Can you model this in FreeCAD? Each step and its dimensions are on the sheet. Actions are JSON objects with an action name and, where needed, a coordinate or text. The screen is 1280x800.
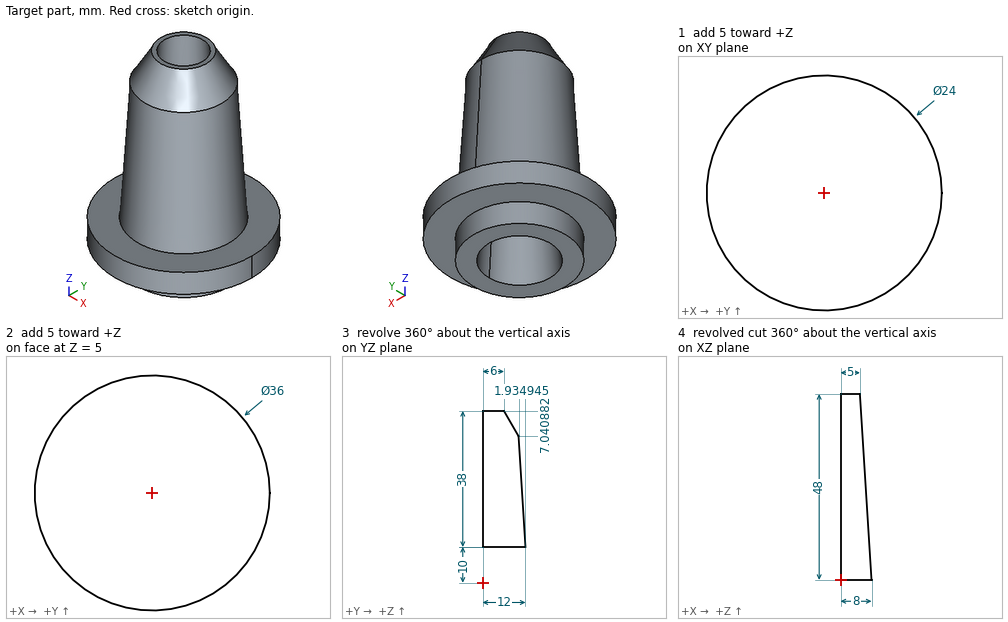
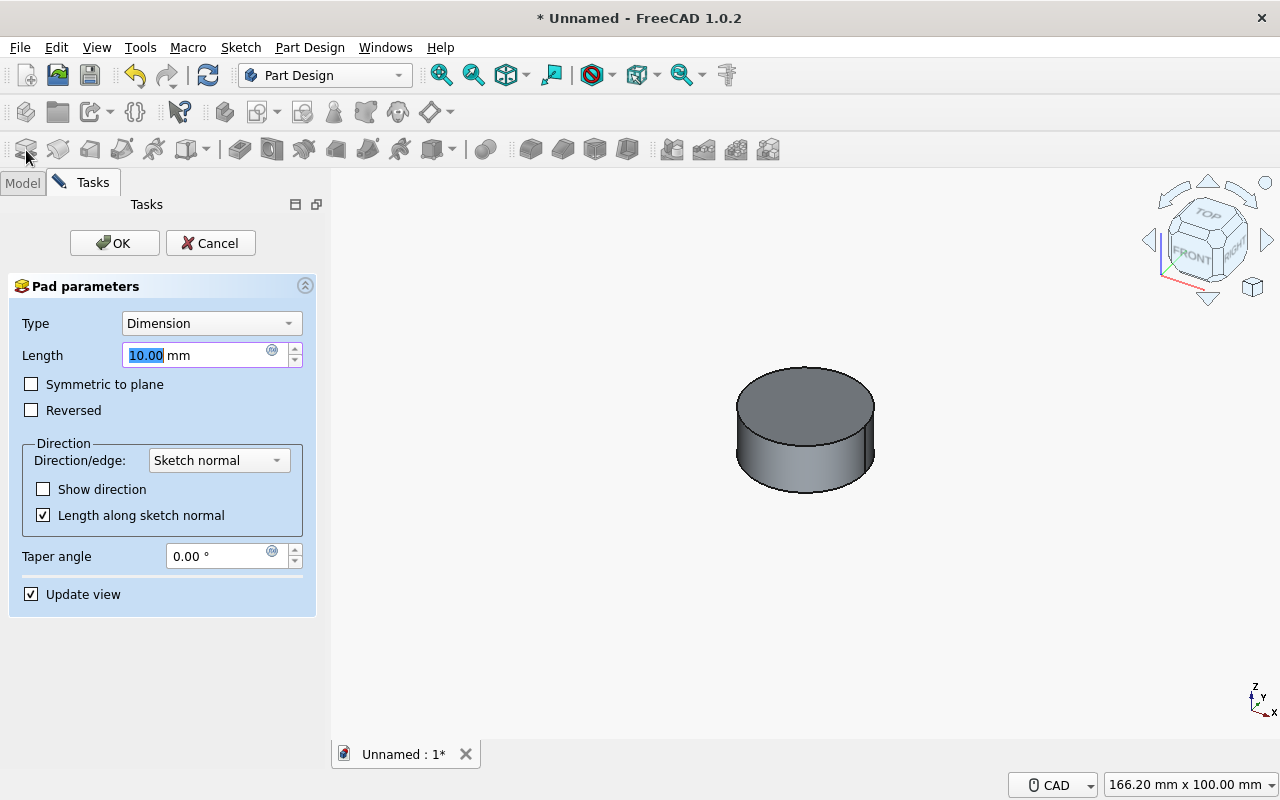
{"action": "type", "text": "5"}
{"action": "key", "text": "Tab"}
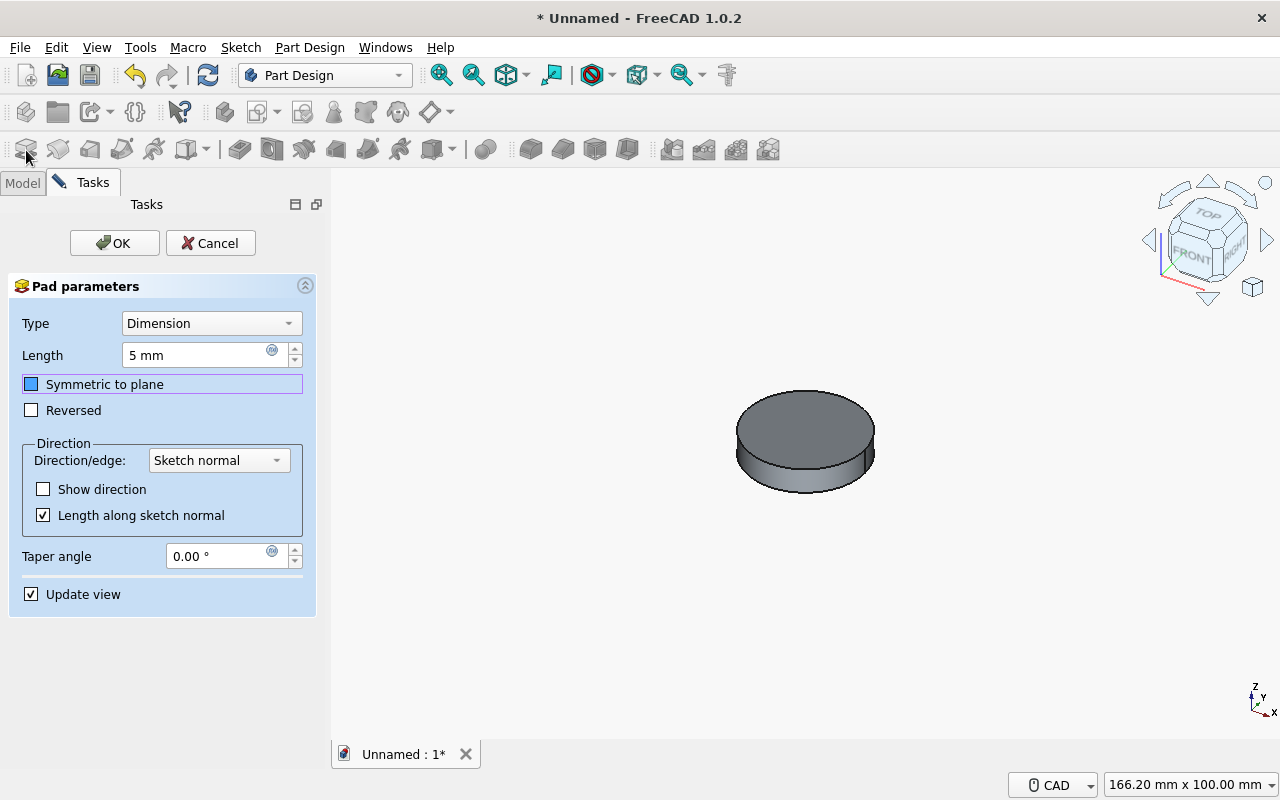
{"action": "left_click", "coordinate": [115, 243]}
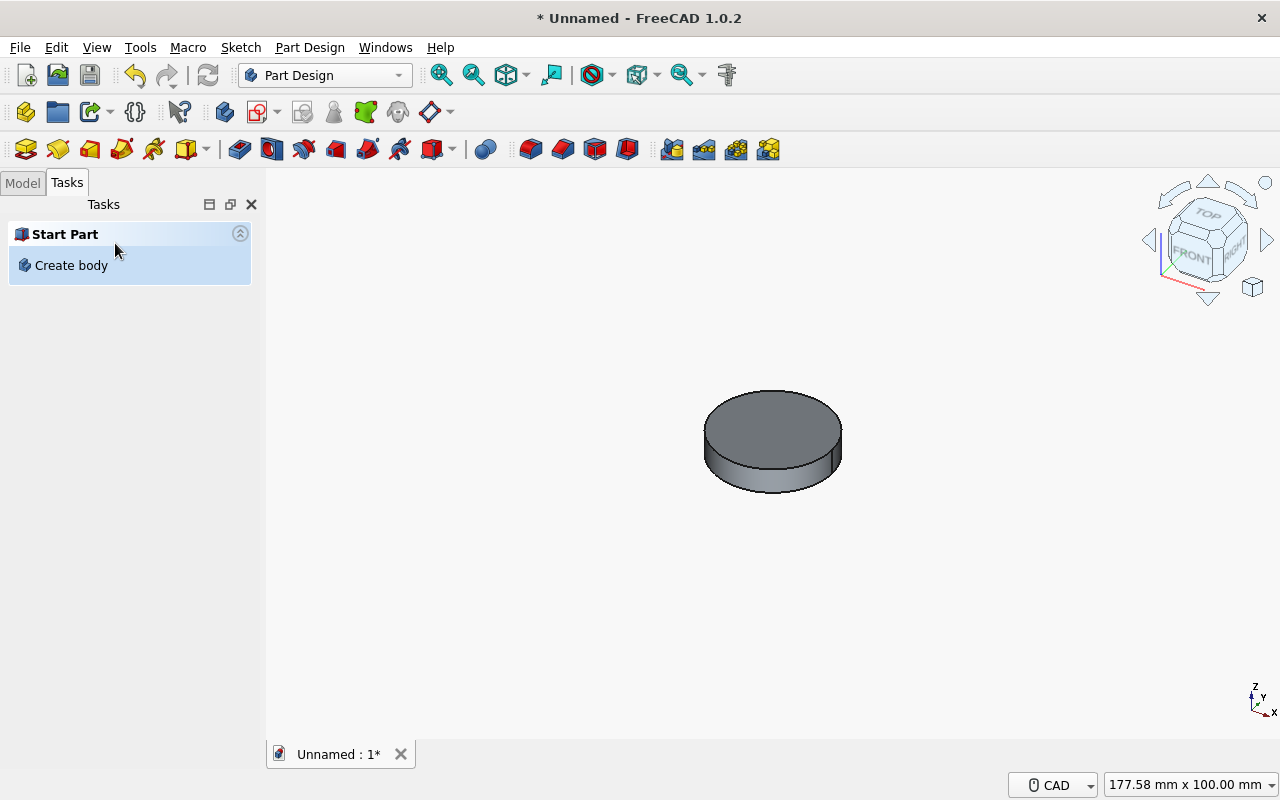
{"action": "left_click", "coordinate": [442, 76]}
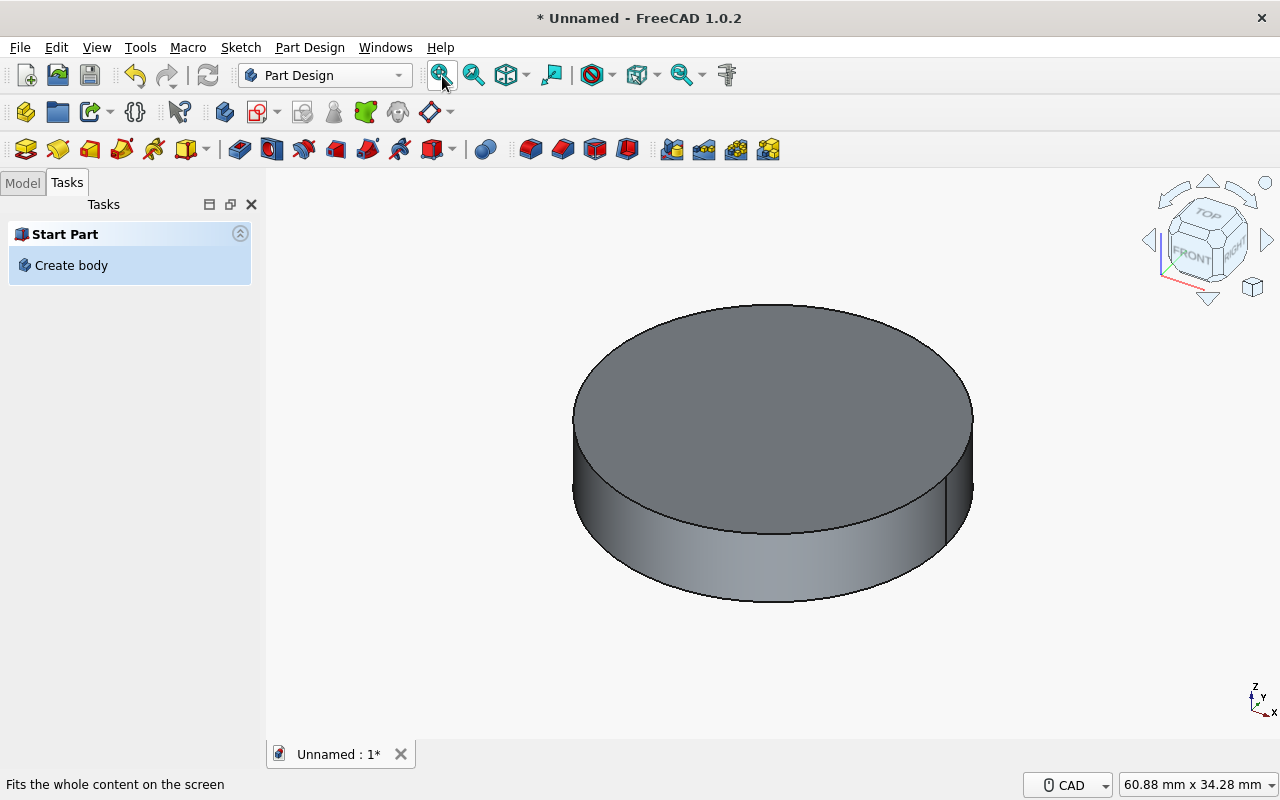
{"action": "left_click", "coordinate": [773, 418]}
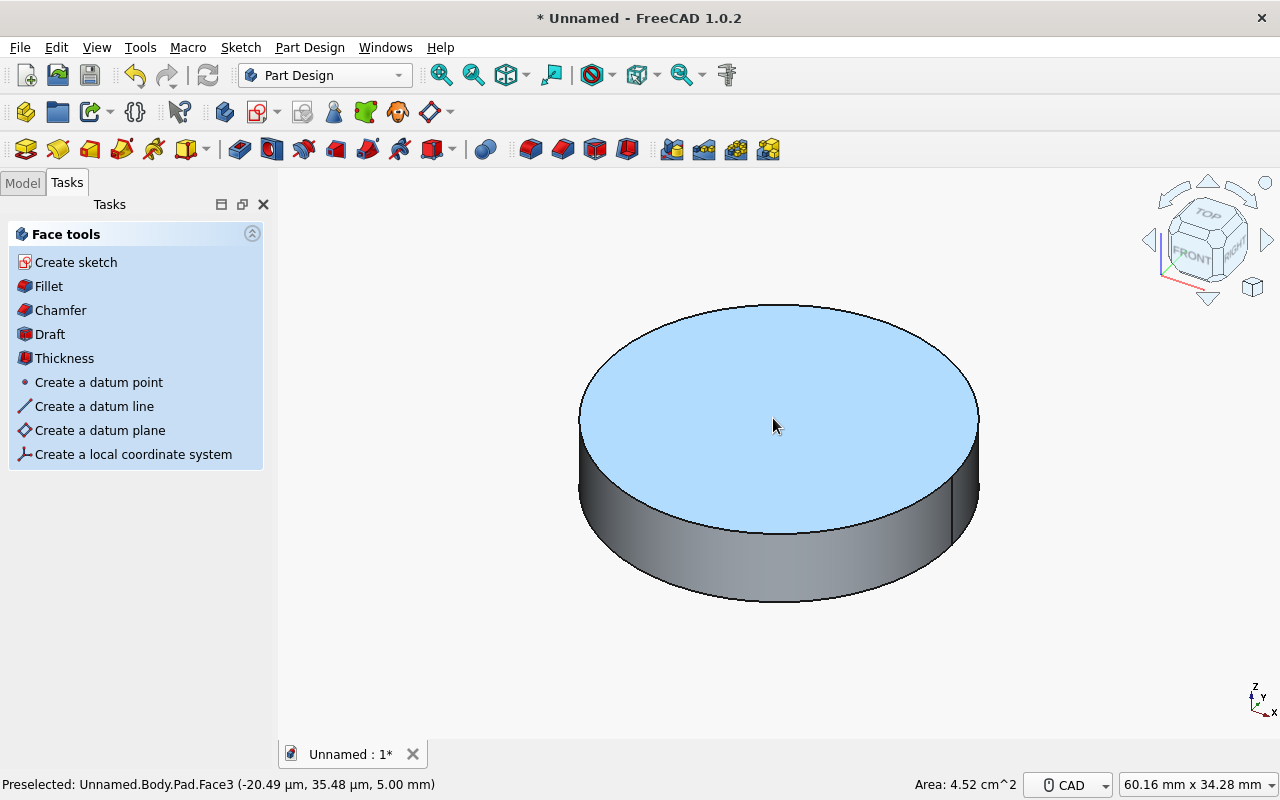
{"action": "left_click", "coordinate": [258, 112]}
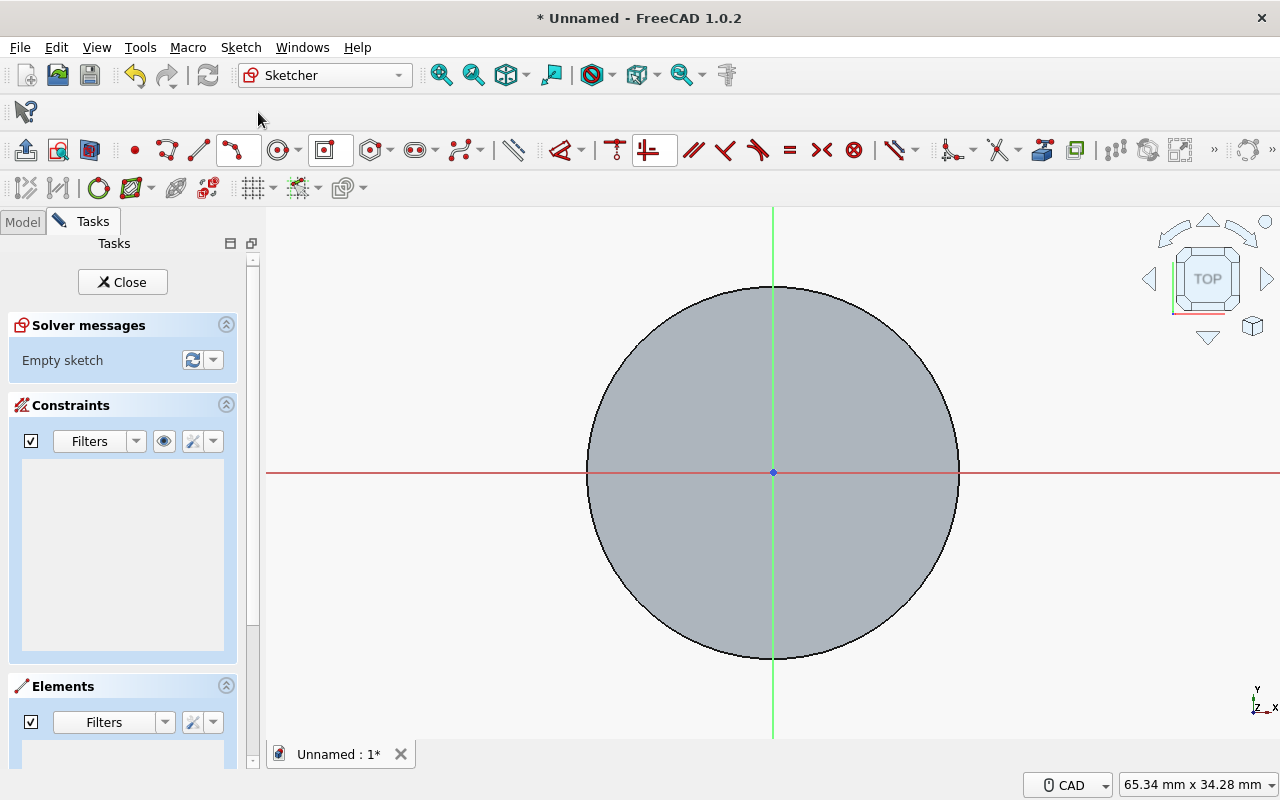
{"action": "scroll", "coordinate": [621, 473], "scroll_direction": "down", "scroll_amount": 3}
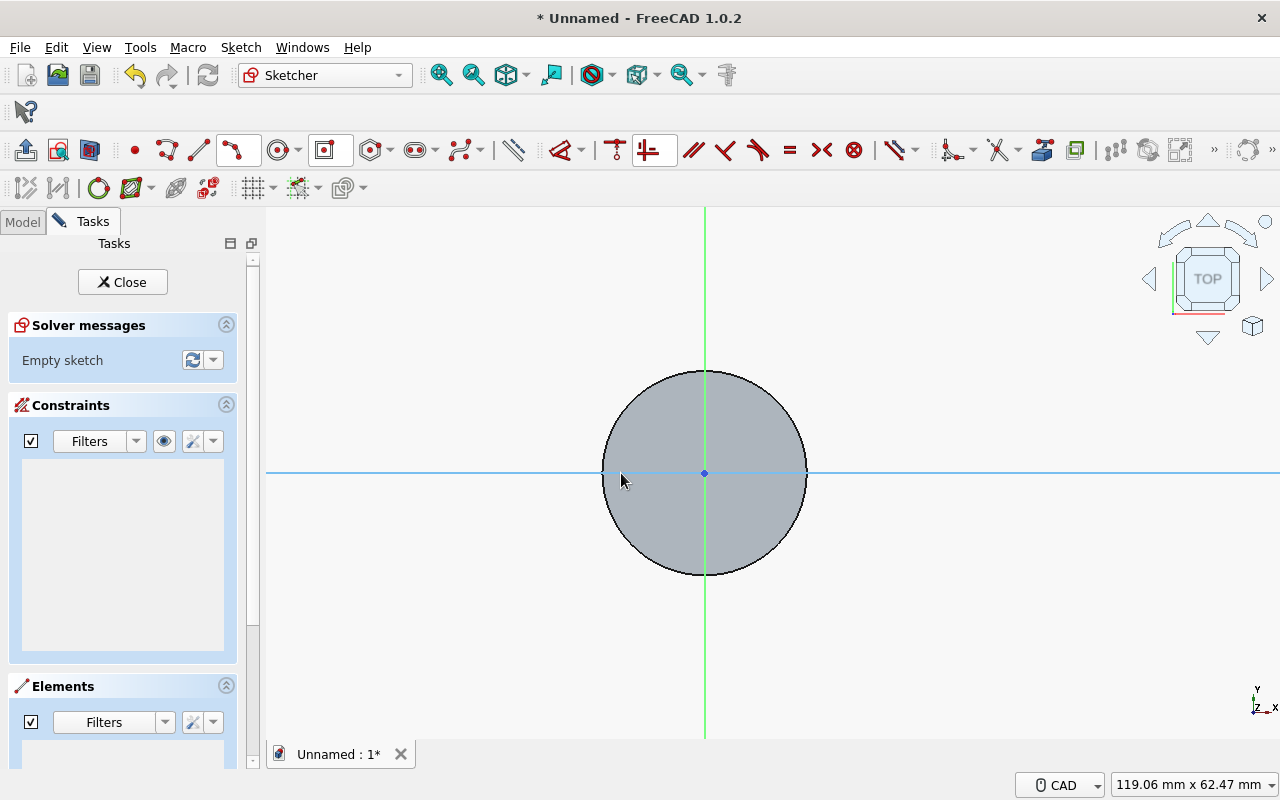
{"action": "left_click", "coordinate": [278, 150]}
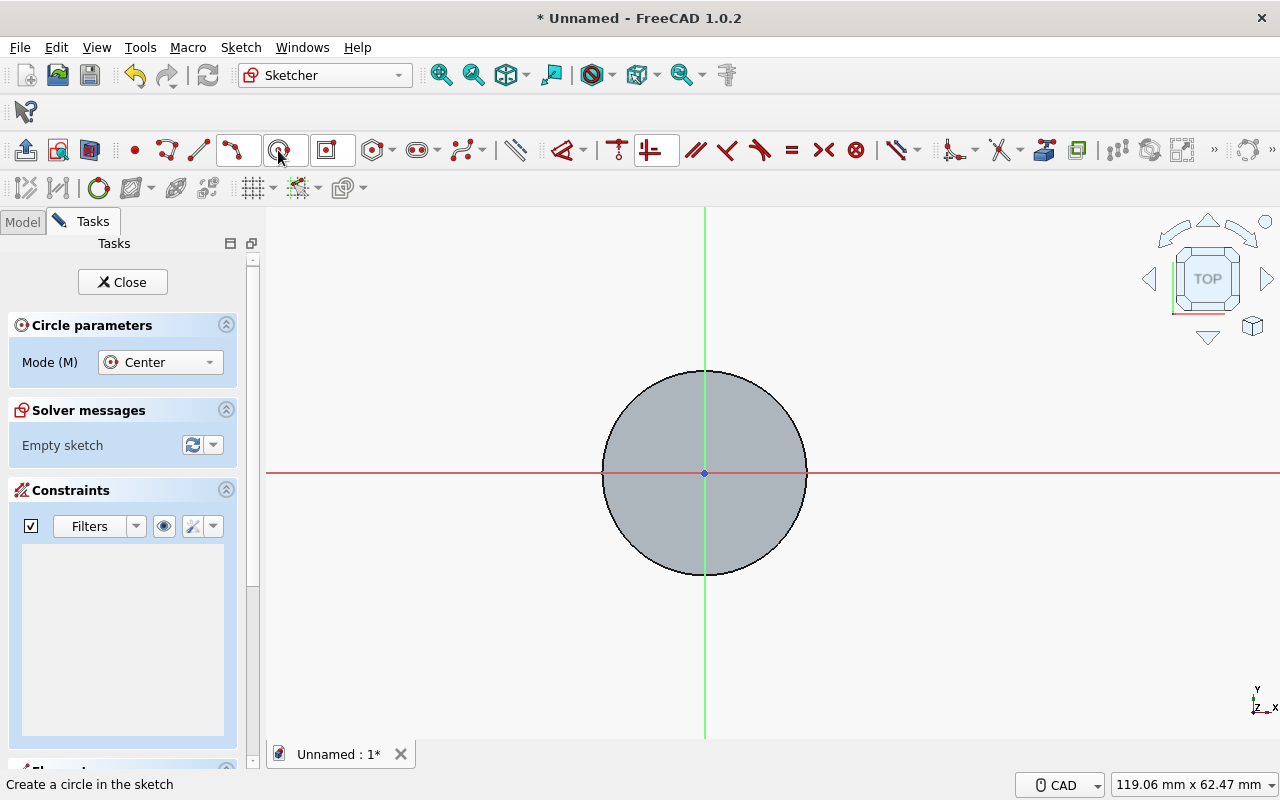
{"action": "left_click", "coordinate": [705, 473]}
{"action": "mouse_move", "coordinate": [813, 365]}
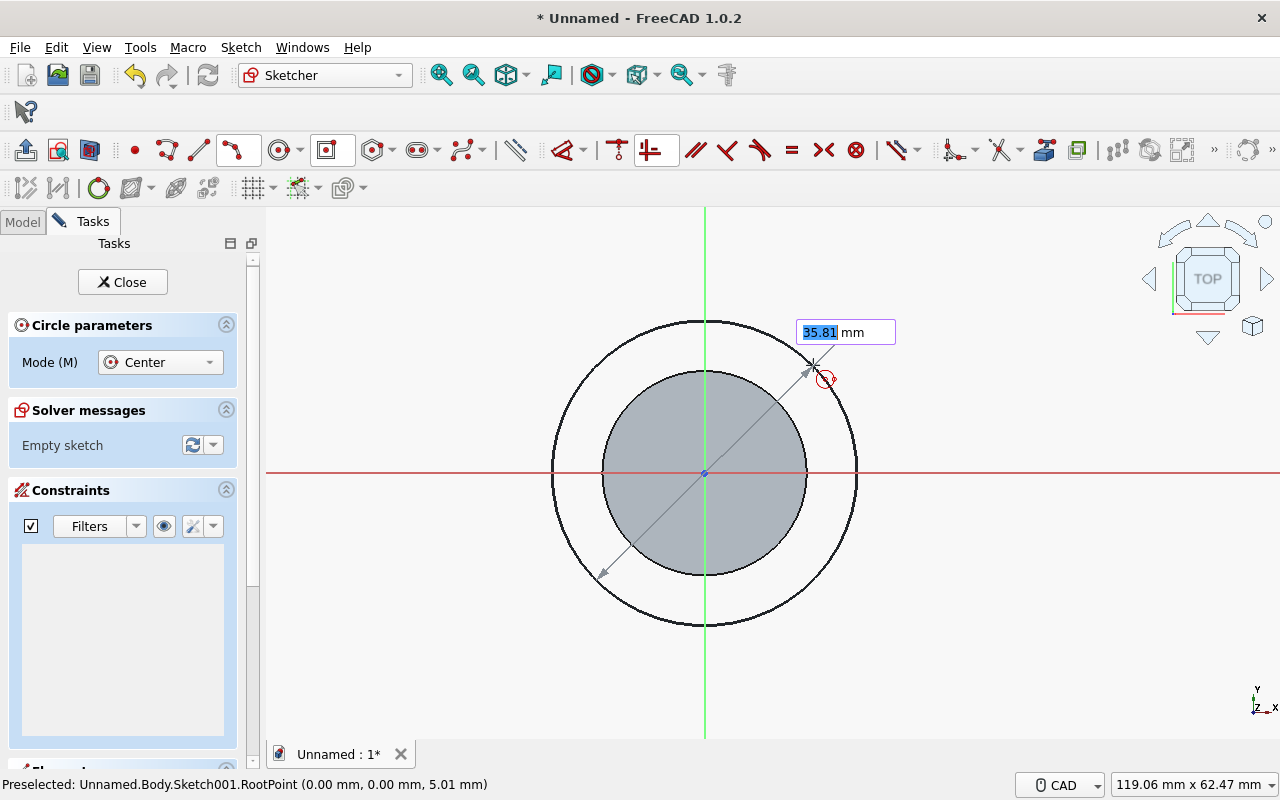
{"action": "type", "text": "36"}
{"action": "key", "text": "Return"}
{"action": "key", "text": "Escape"}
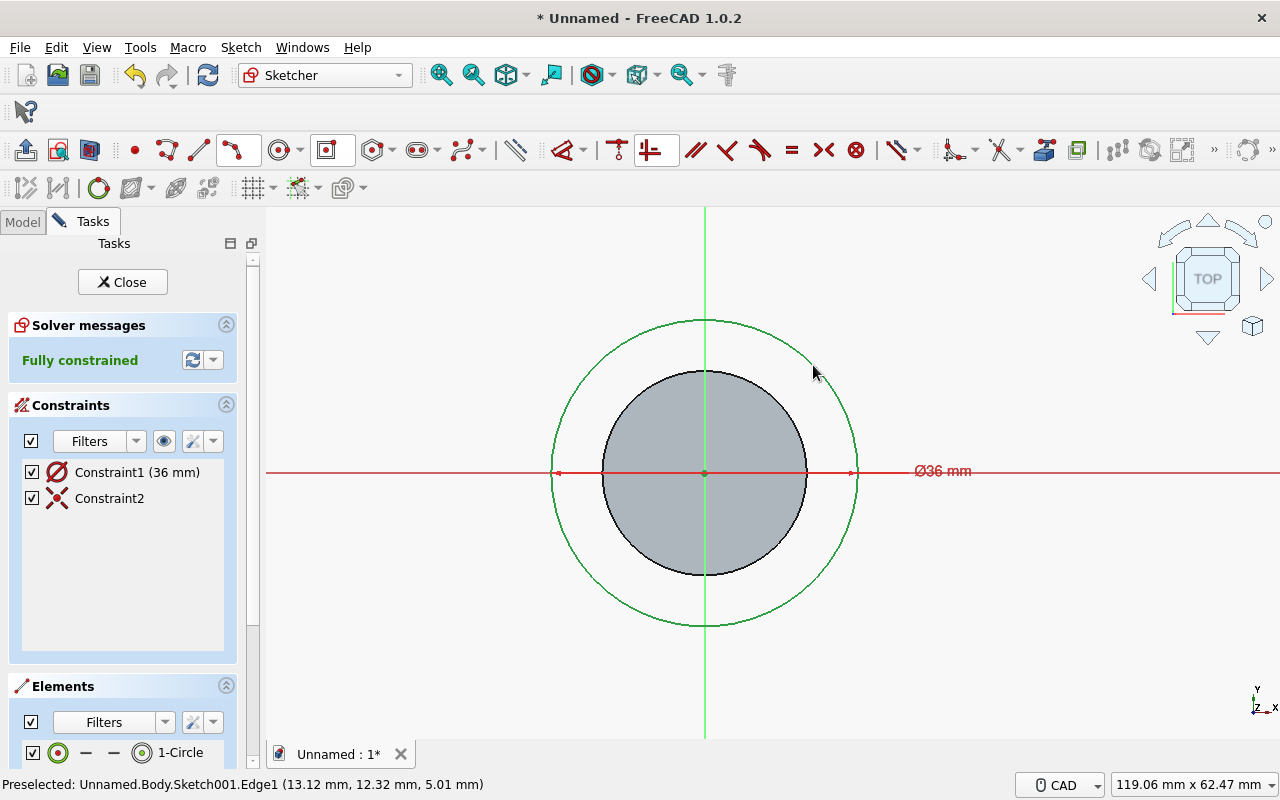
{"action": "left_click", "coordinate": [123, 282]}